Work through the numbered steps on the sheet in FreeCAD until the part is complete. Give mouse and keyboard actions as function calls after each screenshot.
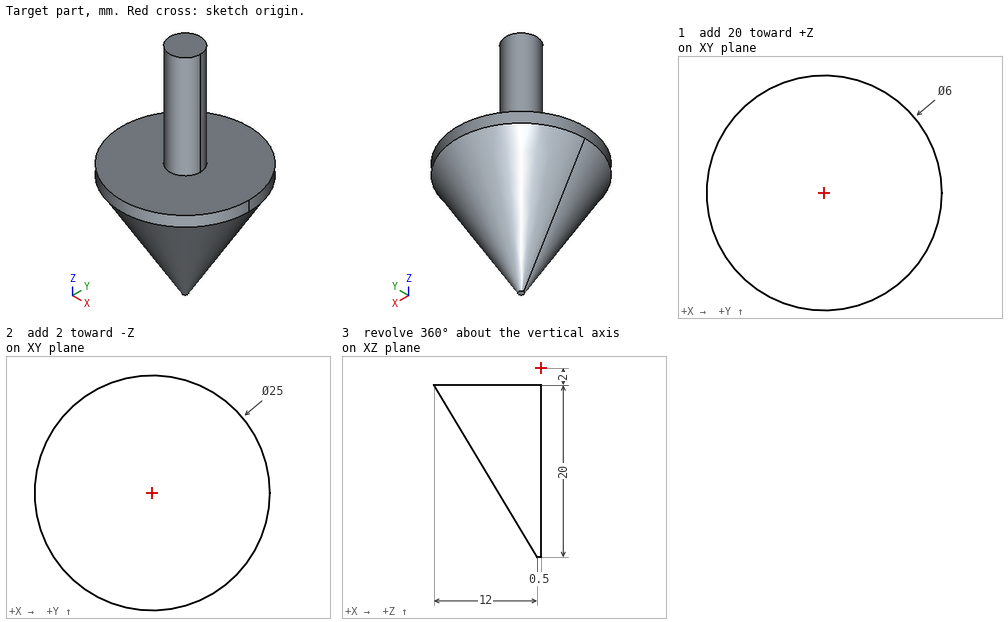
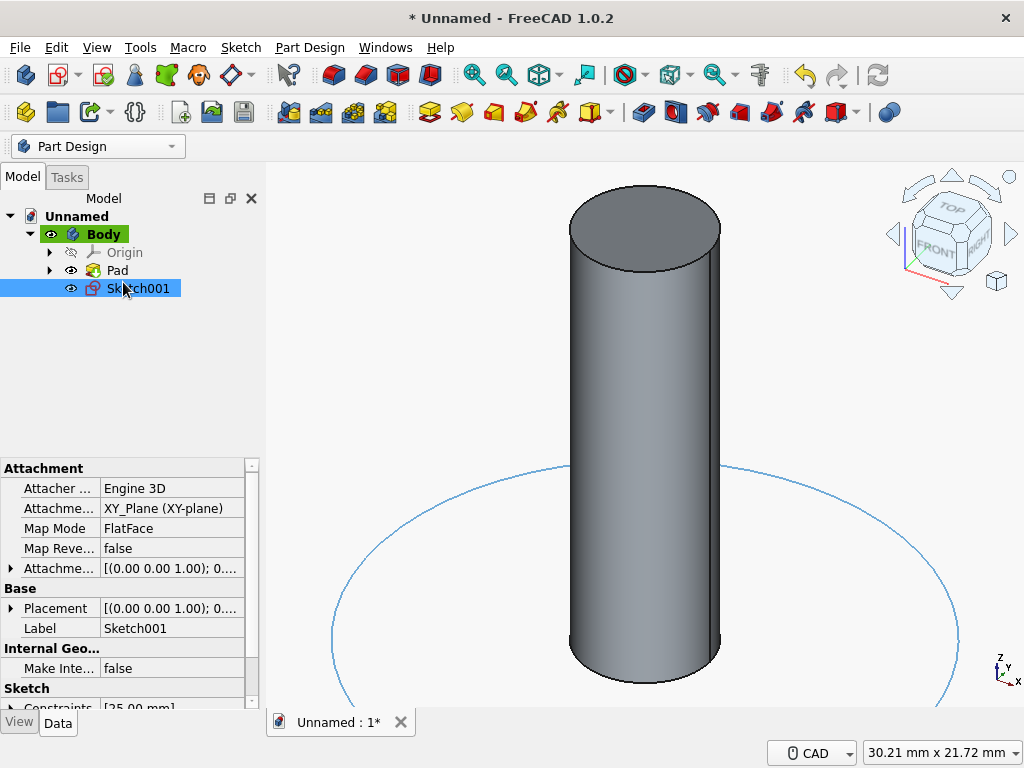
click(430, 112)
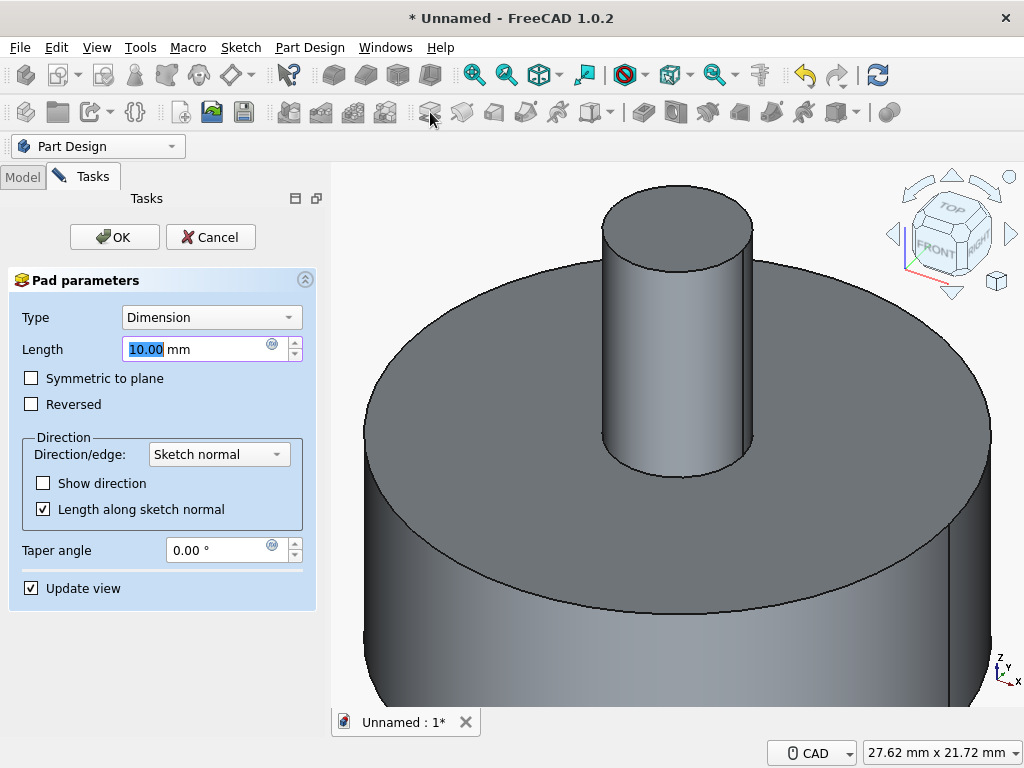
text(2)
key(Tab)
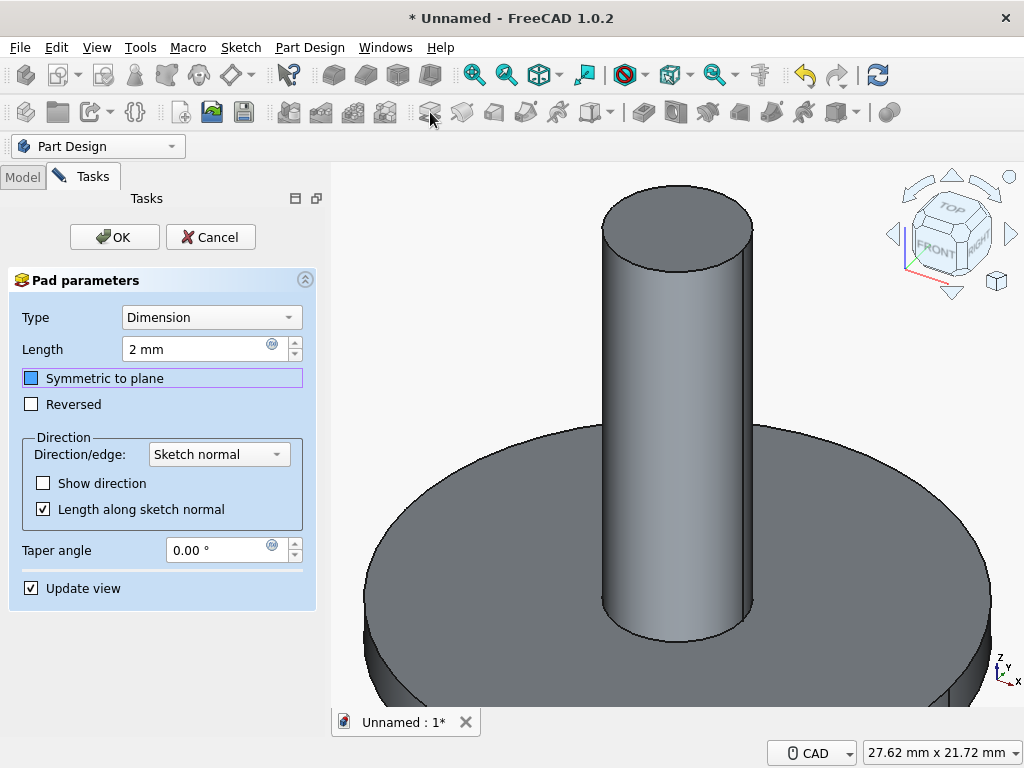
click(30, 404)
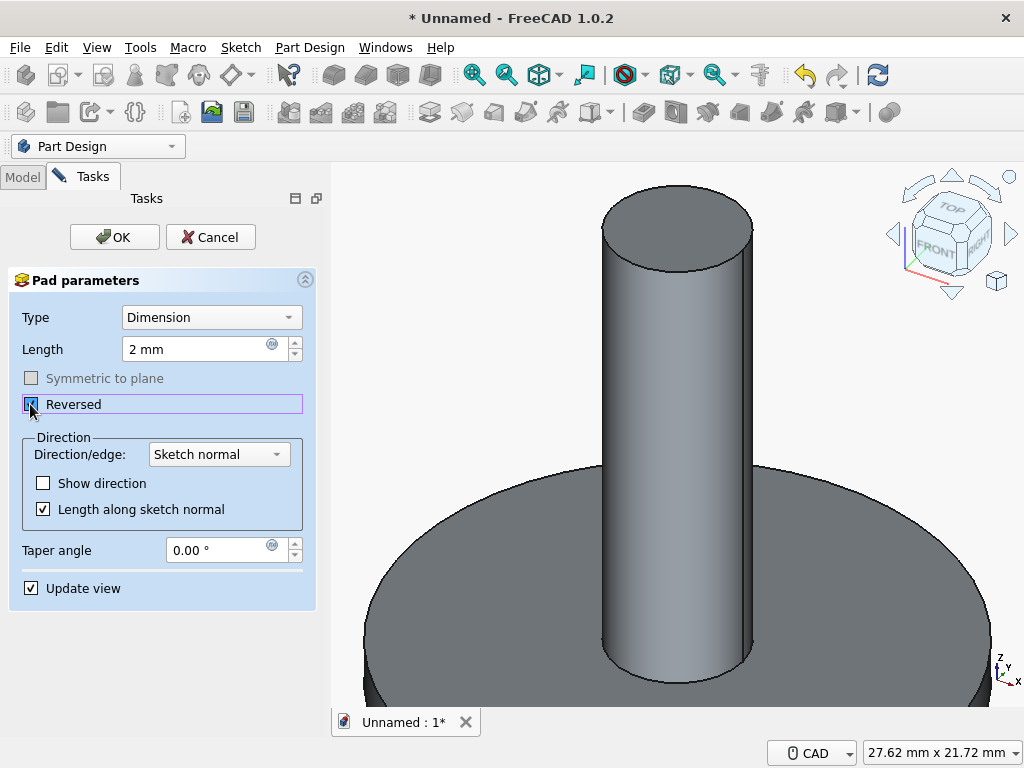
click(115, 237)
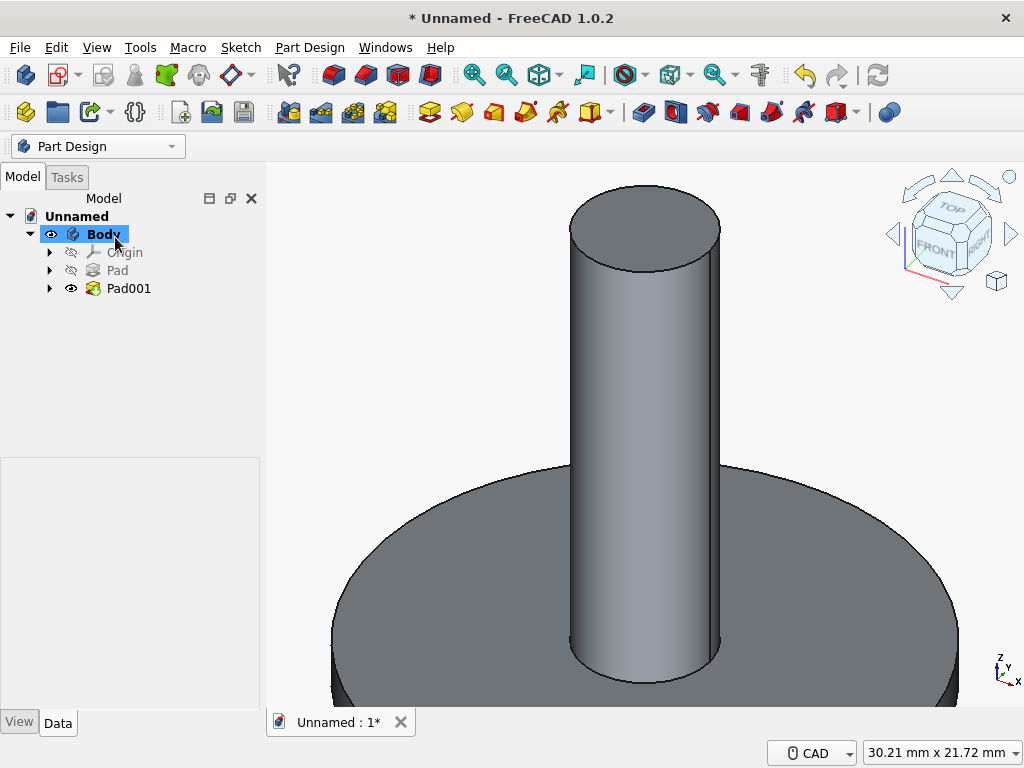
click(476, 76)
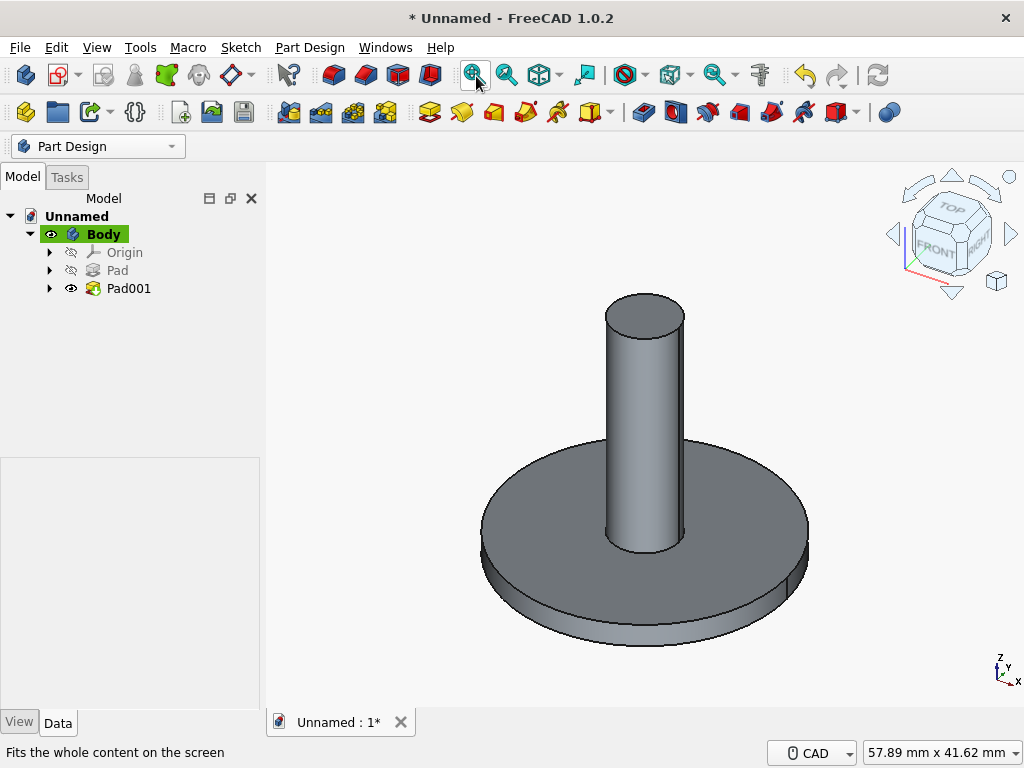
click(58, 76)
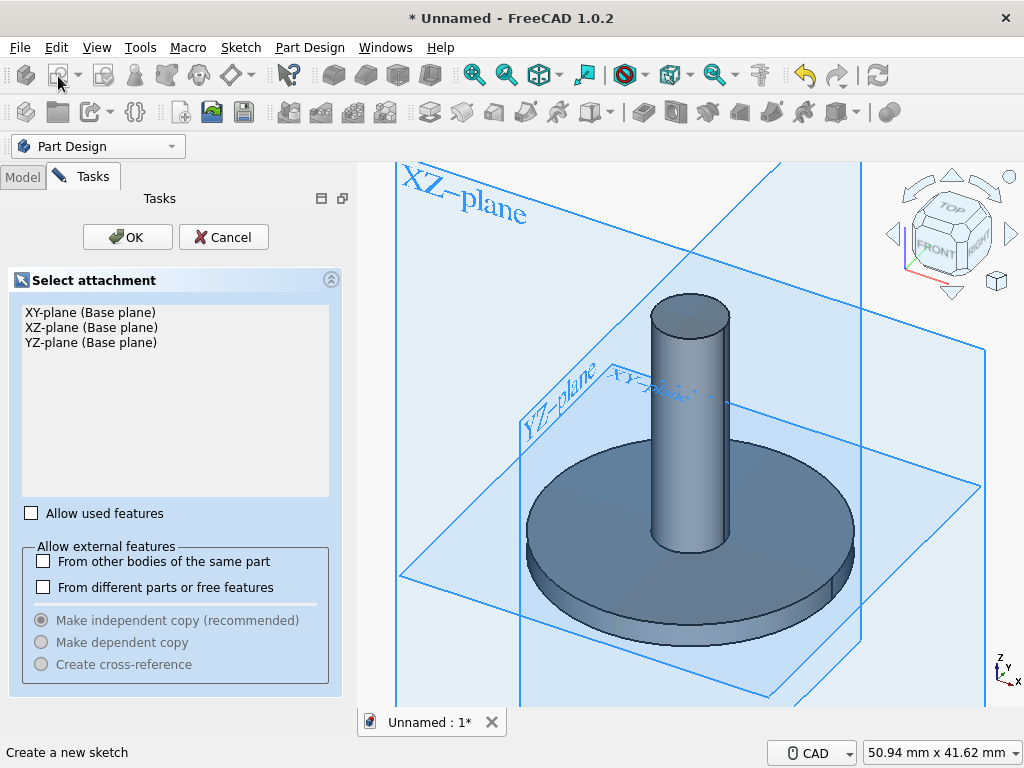
click(82, 328)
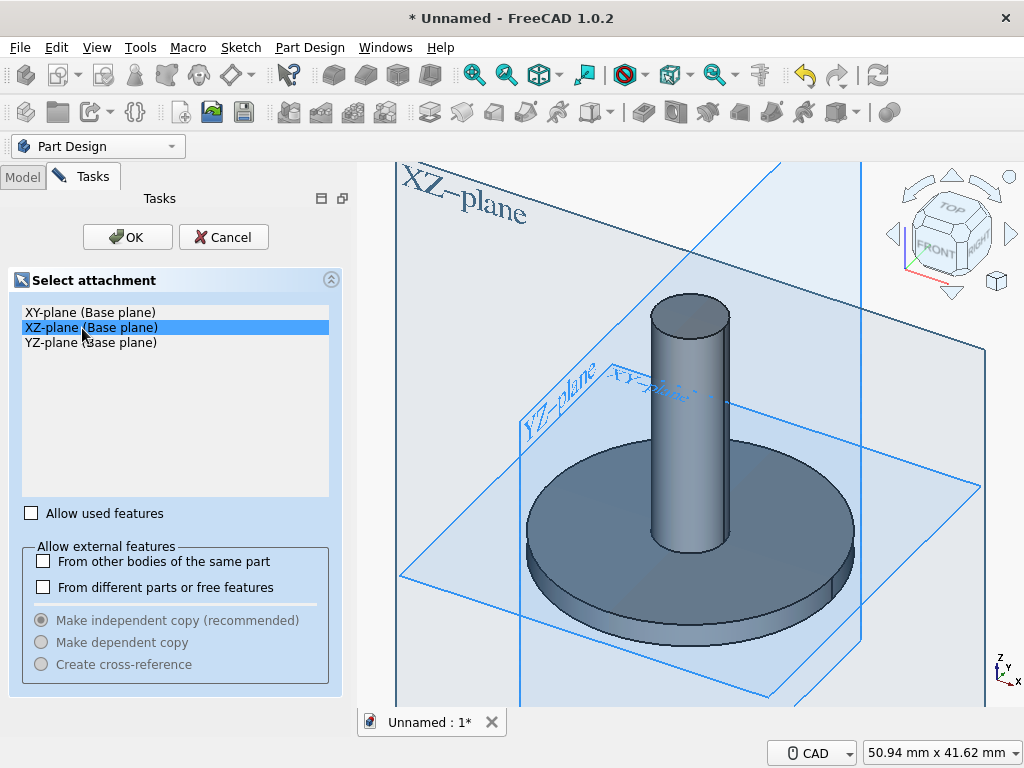
click(128, 237)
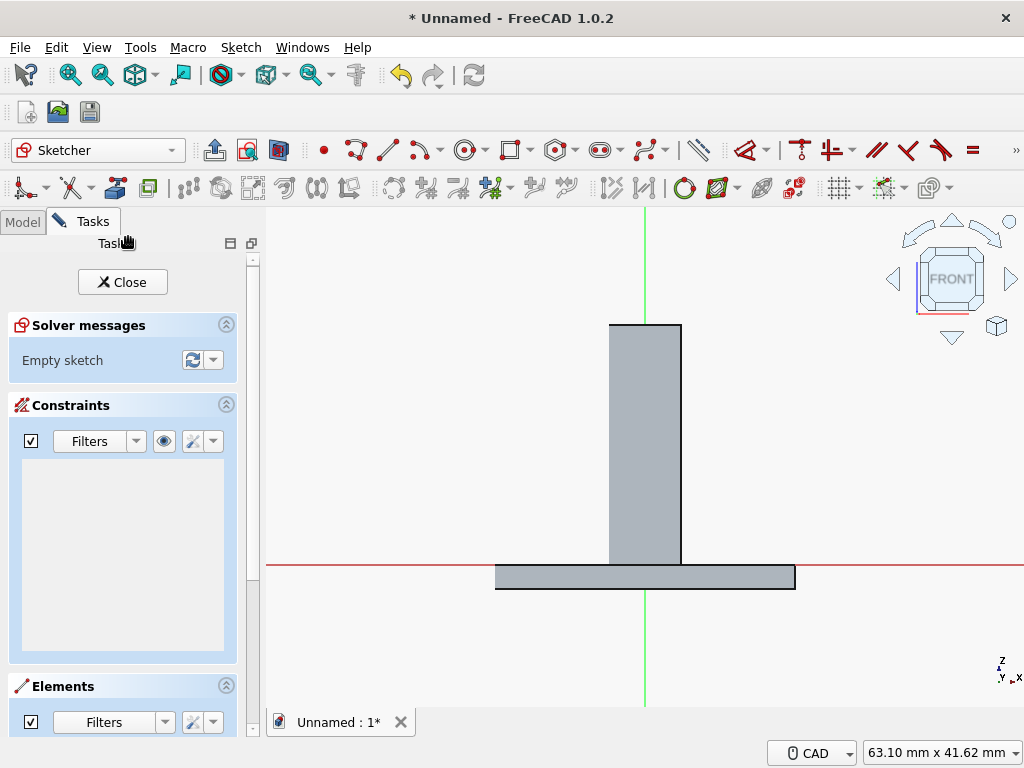
click(280, 150)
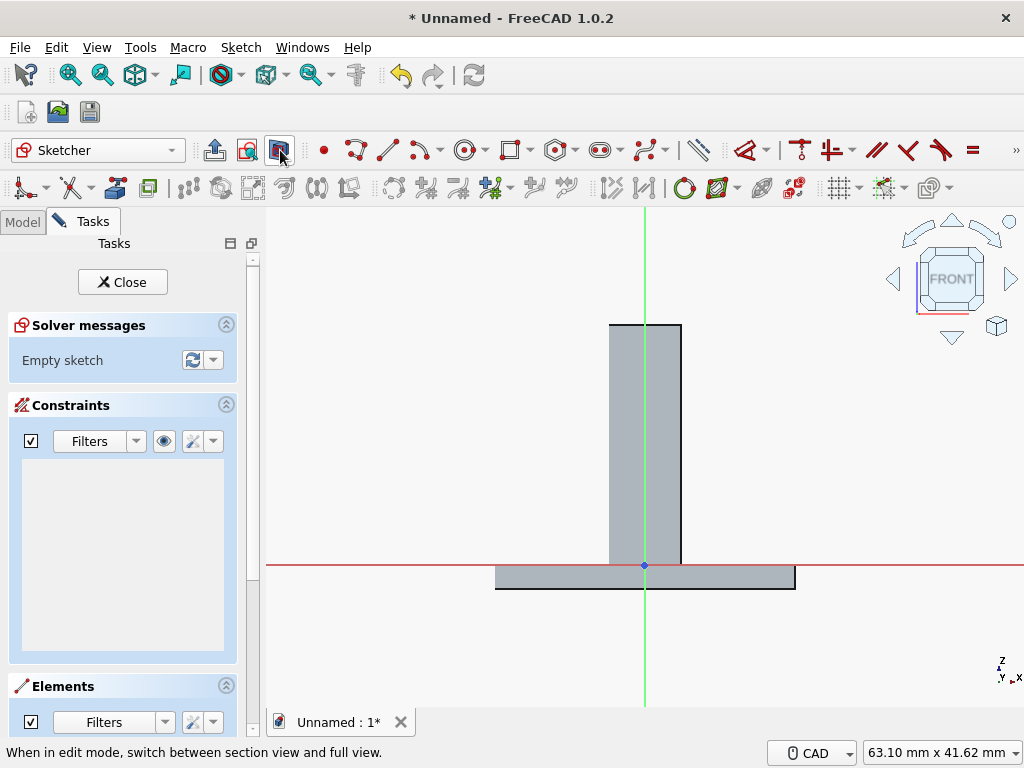
scroll(590, 235, down, 2)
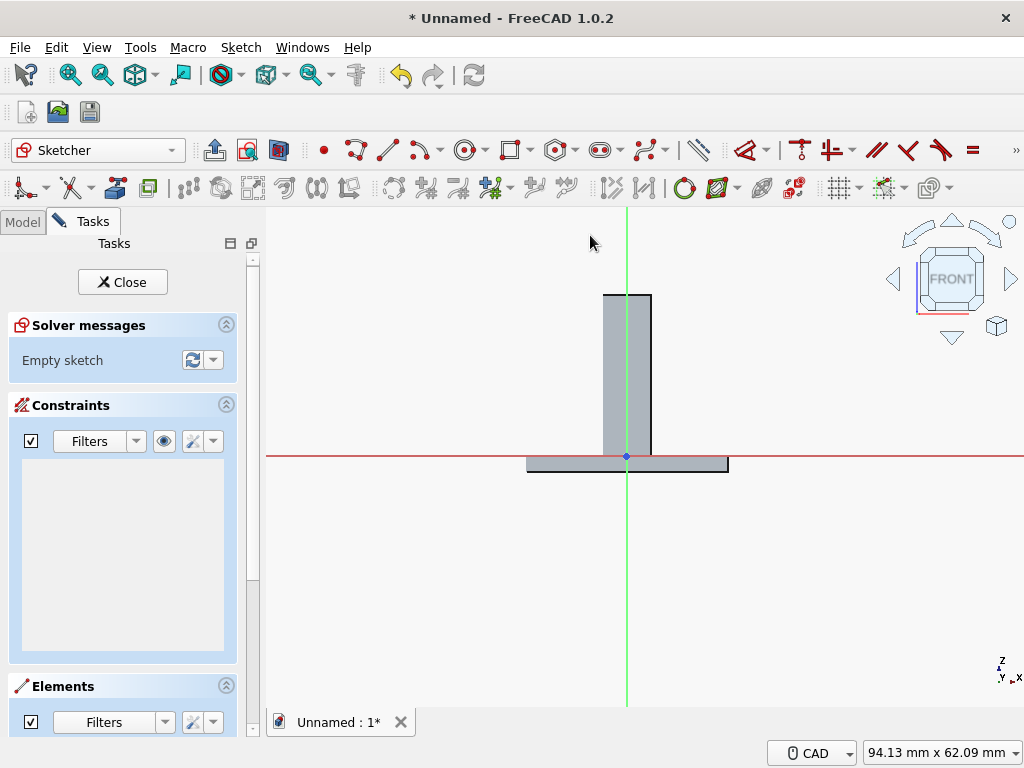
scroll(577, 652, up, 3)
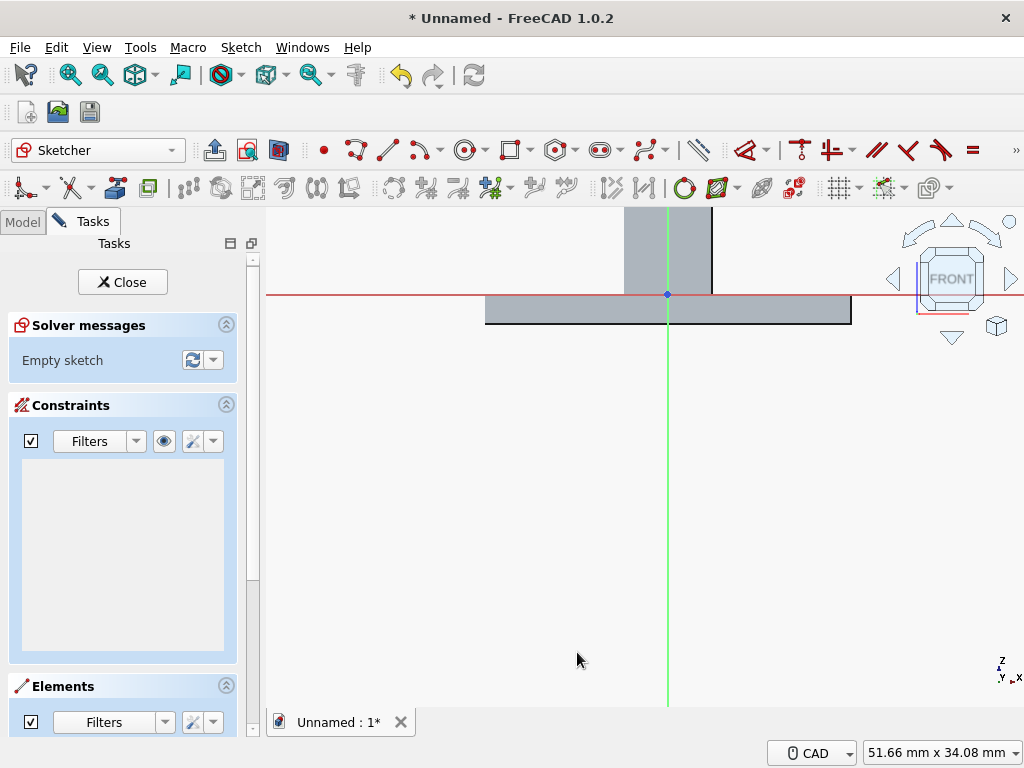
click(356, 150)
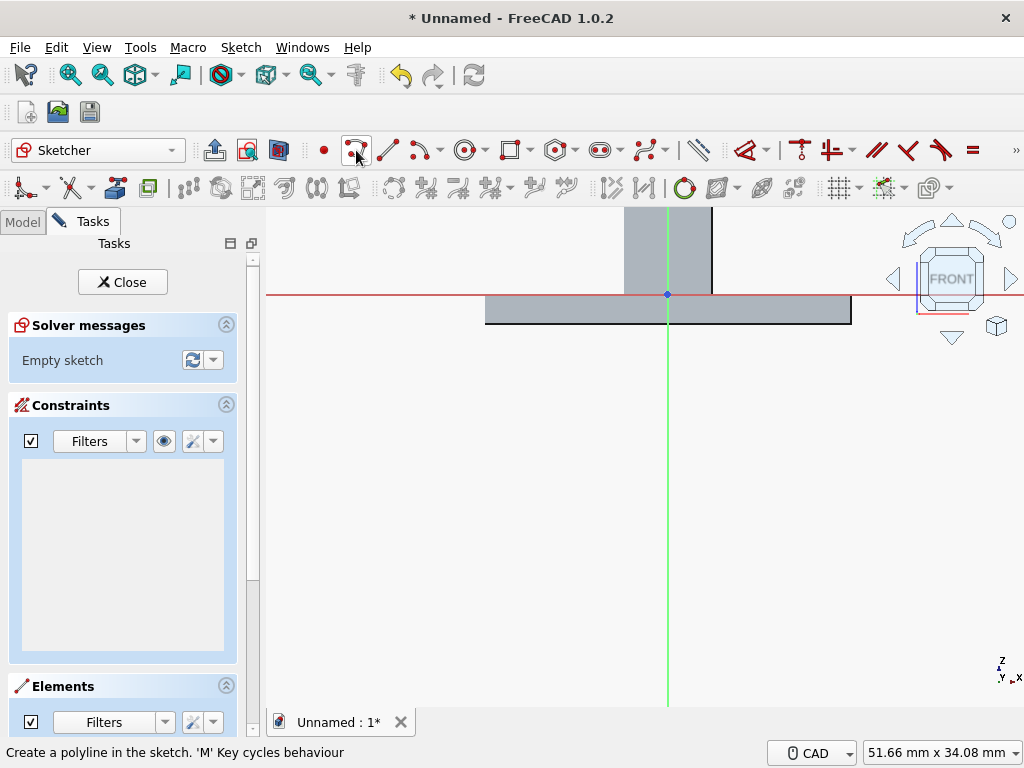
click(668, 324)
click(659, 617)